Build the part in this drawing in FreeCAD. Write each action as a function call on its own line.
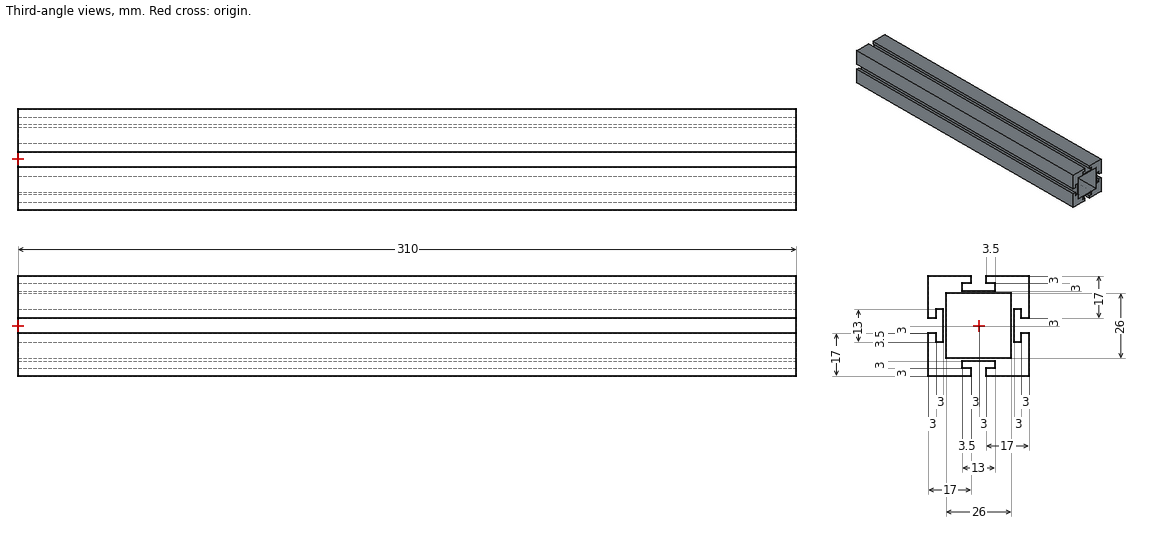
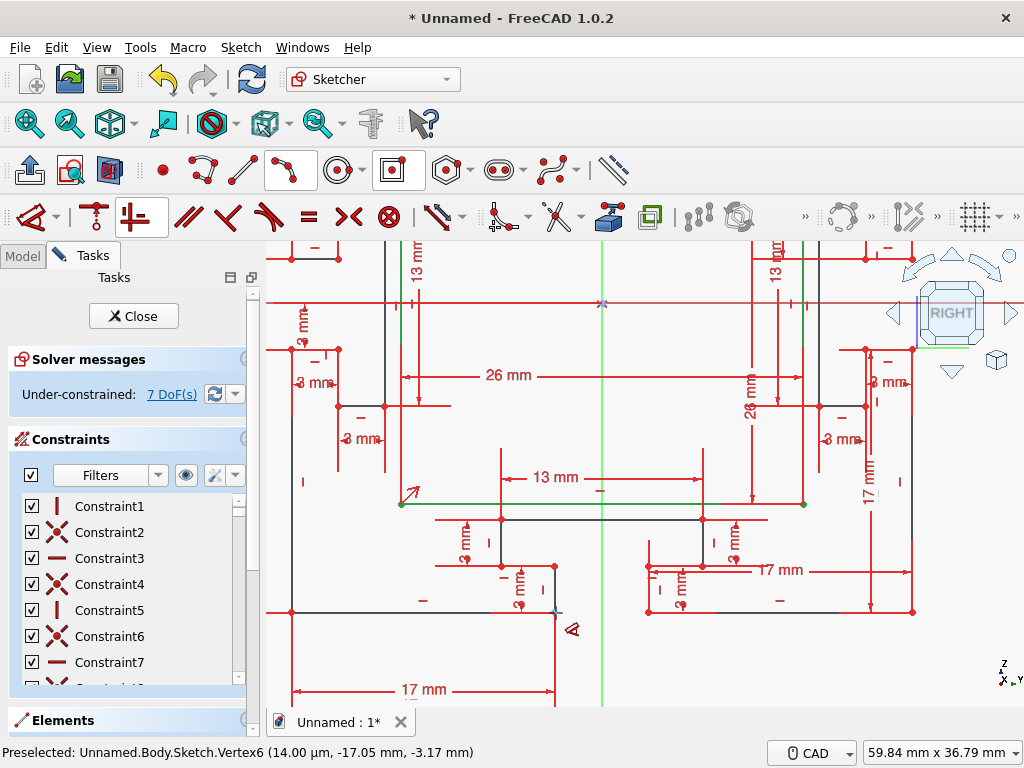
click(555, 613)
click(579, 647)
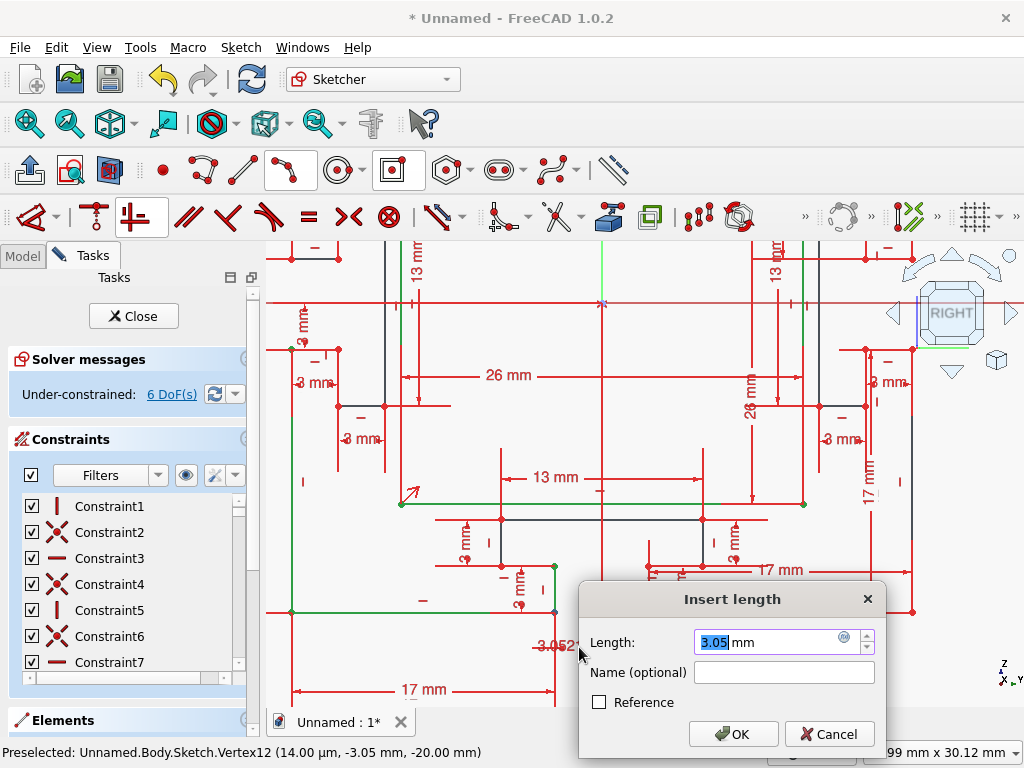
text(3)
key(Return)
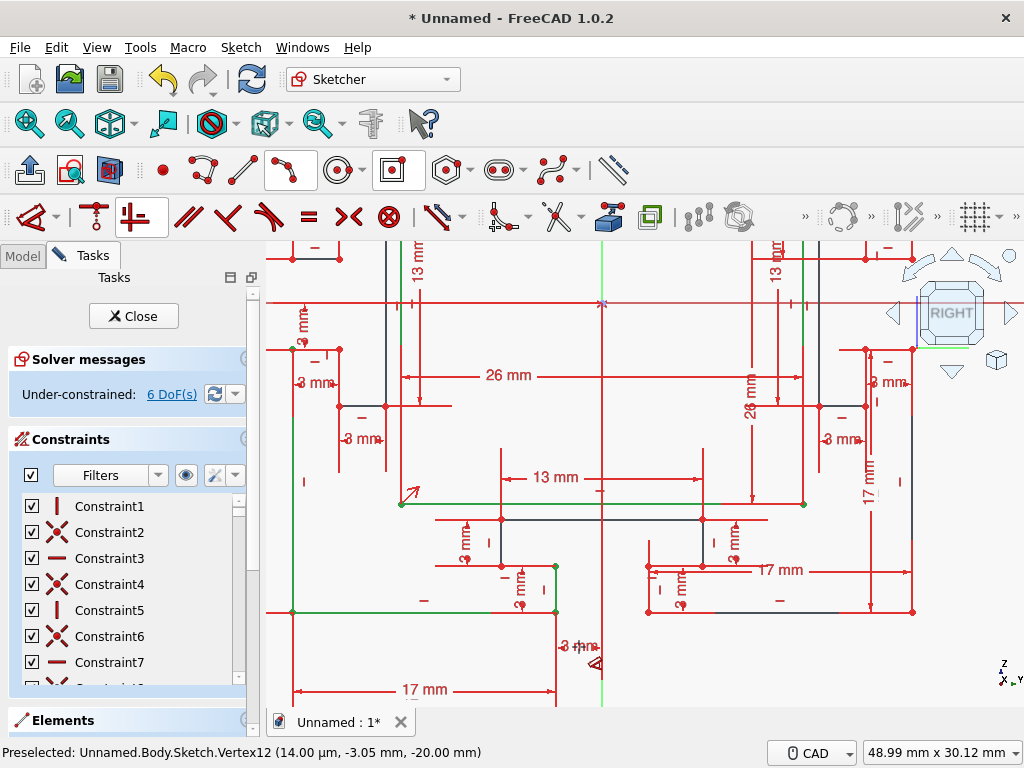
click(649, 566)
click(626, 269)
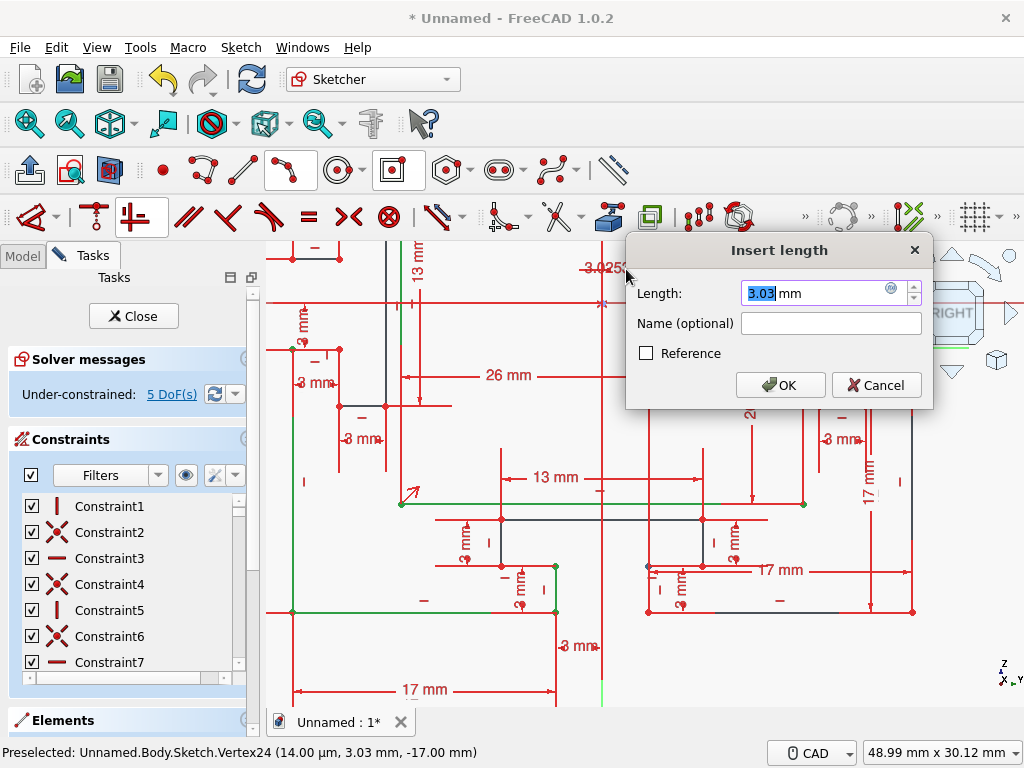
text(3)
key(Return)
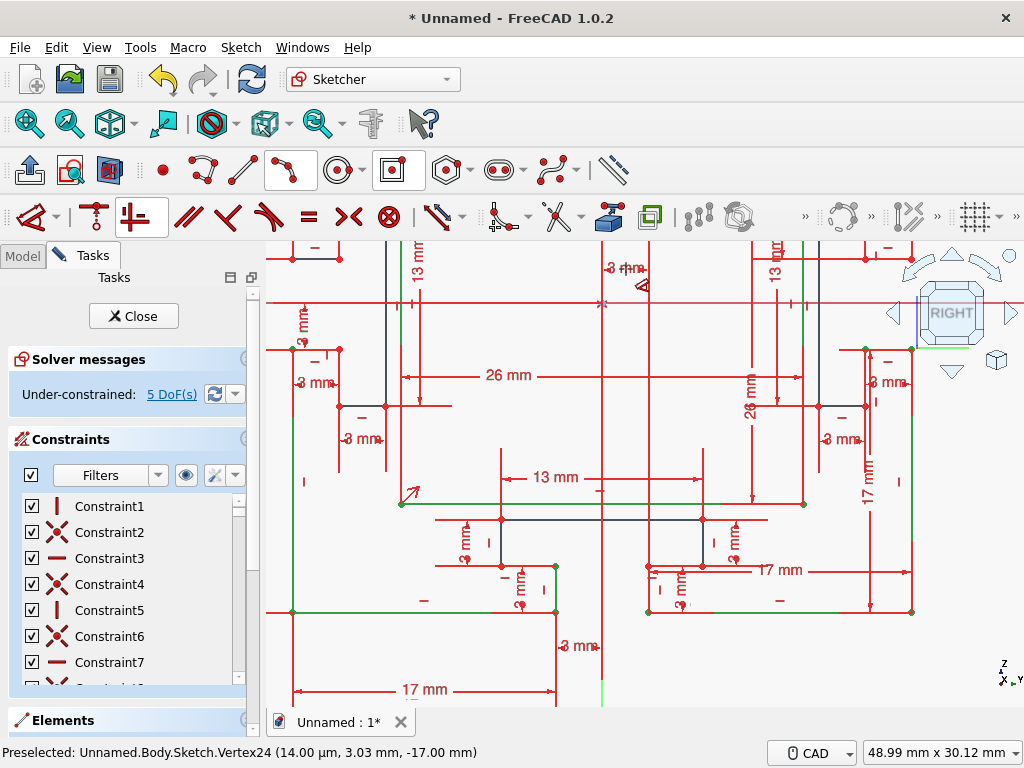
scroll(556, 613, down, 4)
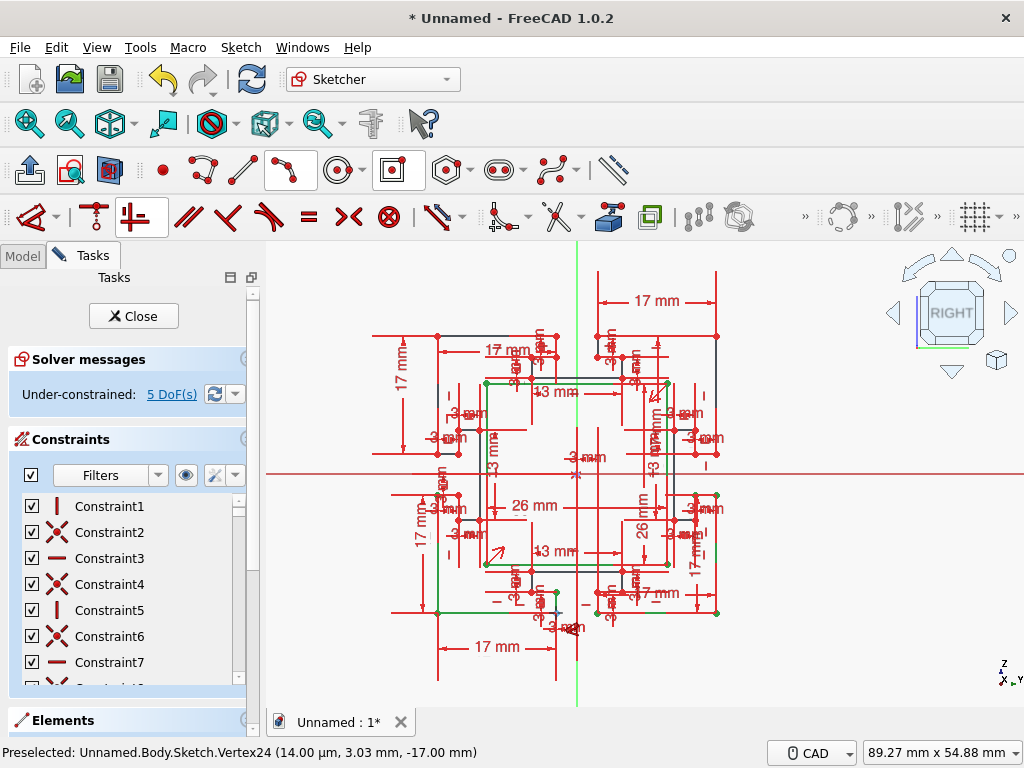
scroll(695, 454, up, 4)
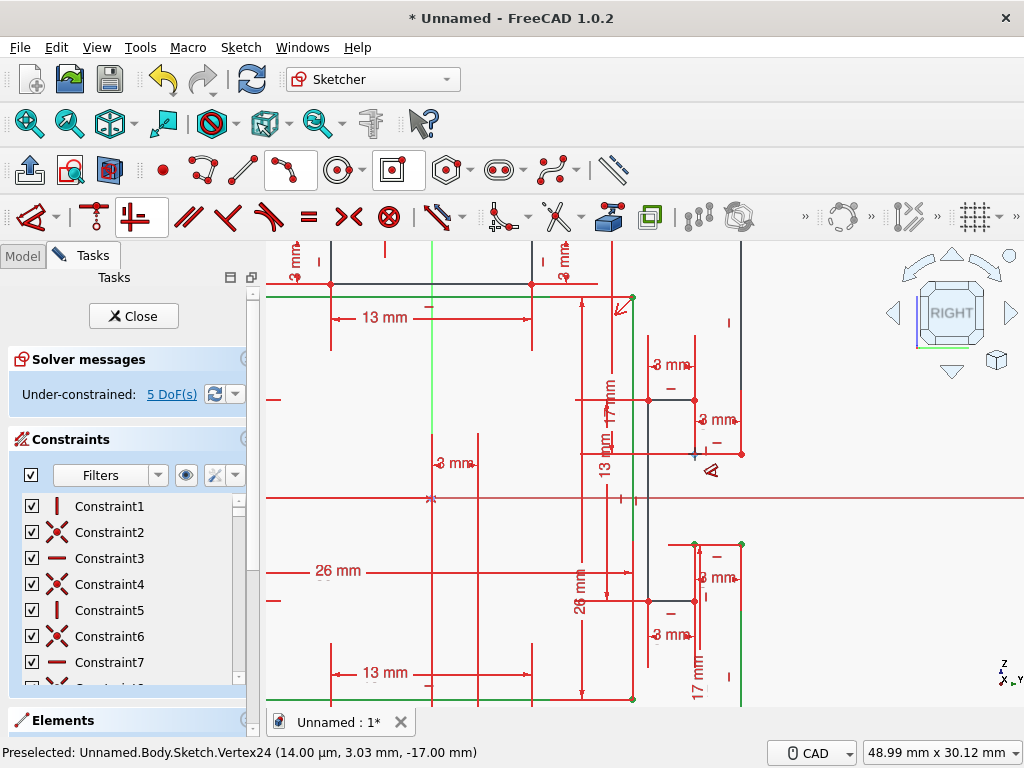
click(695, 454)
click(729, 476)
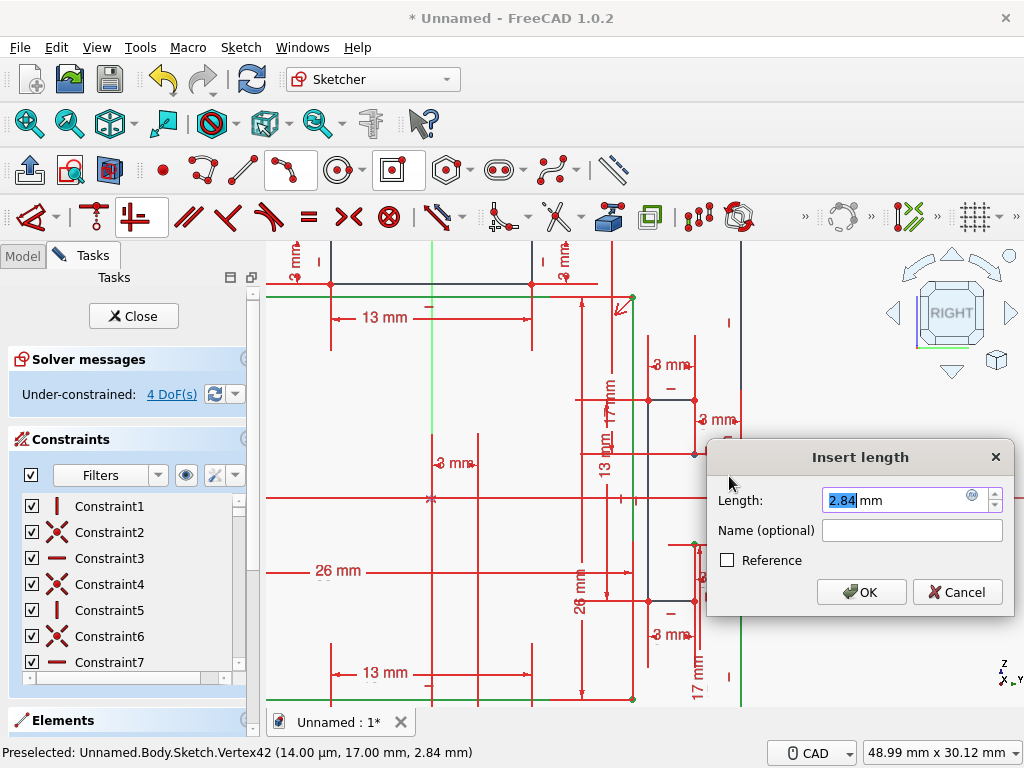
text(3)
key(Return)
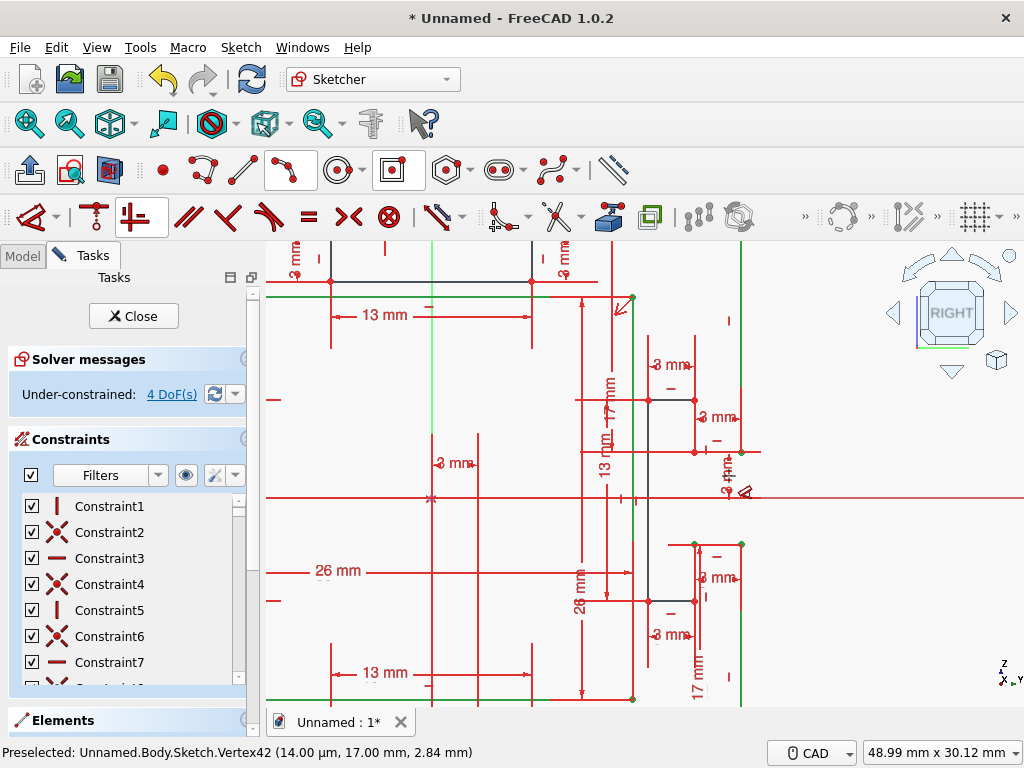
scroll(695, 454, down, 4)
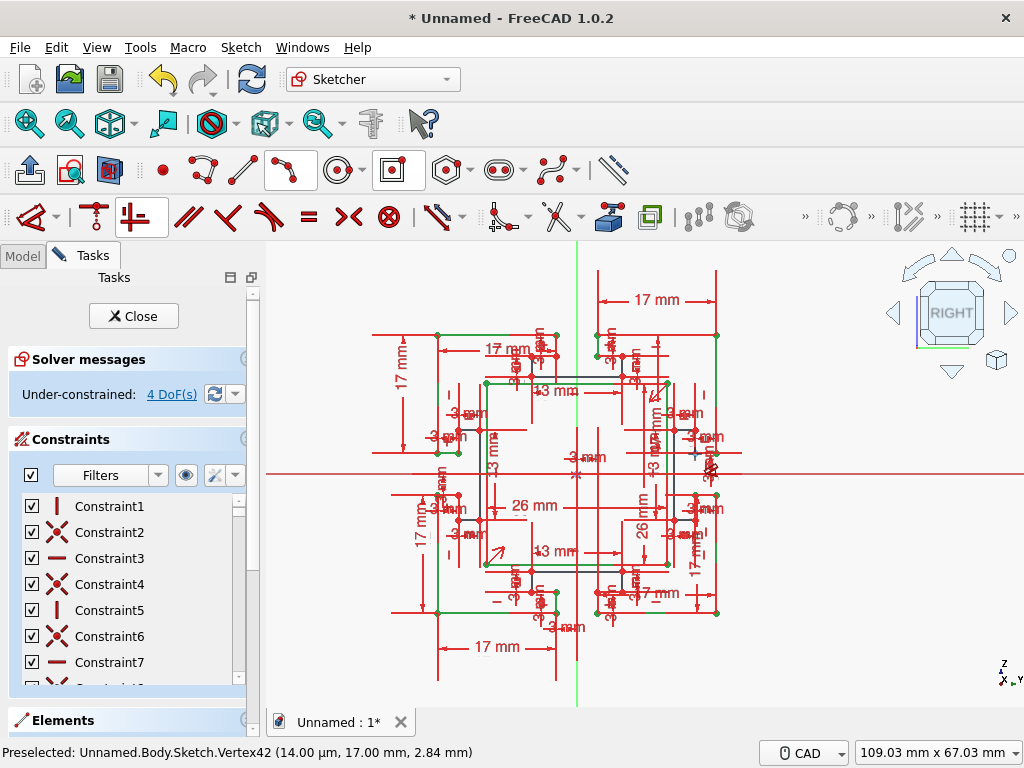
scroll(459, 513, up, 3)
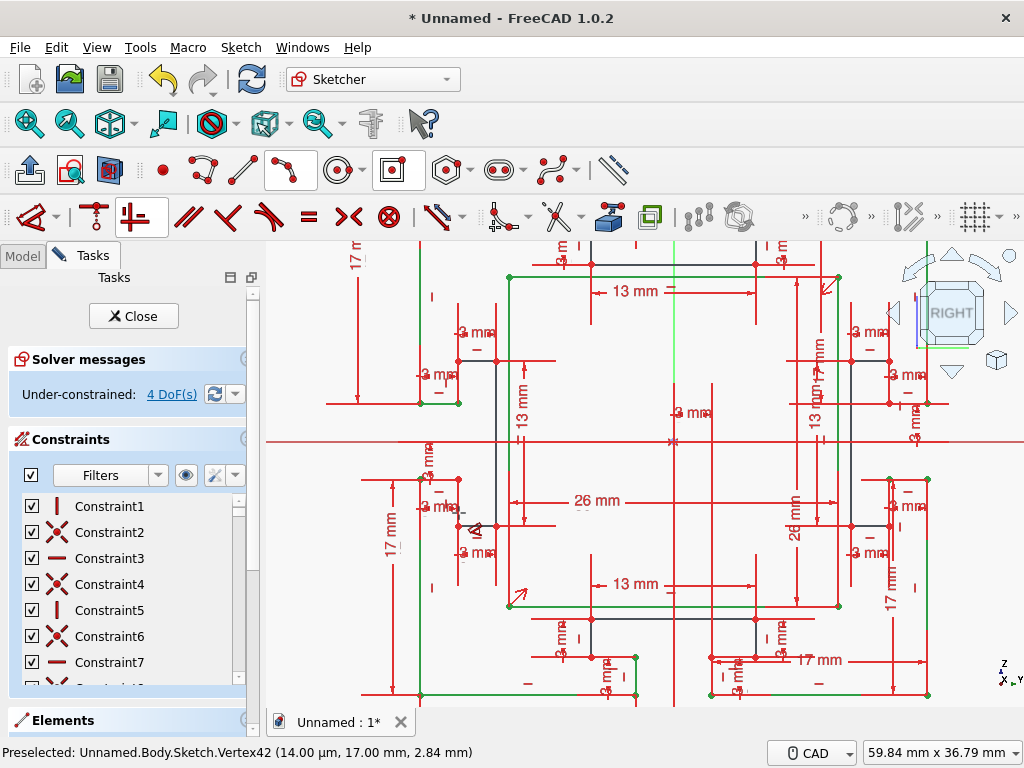
click(458, 512)
click(400, 487)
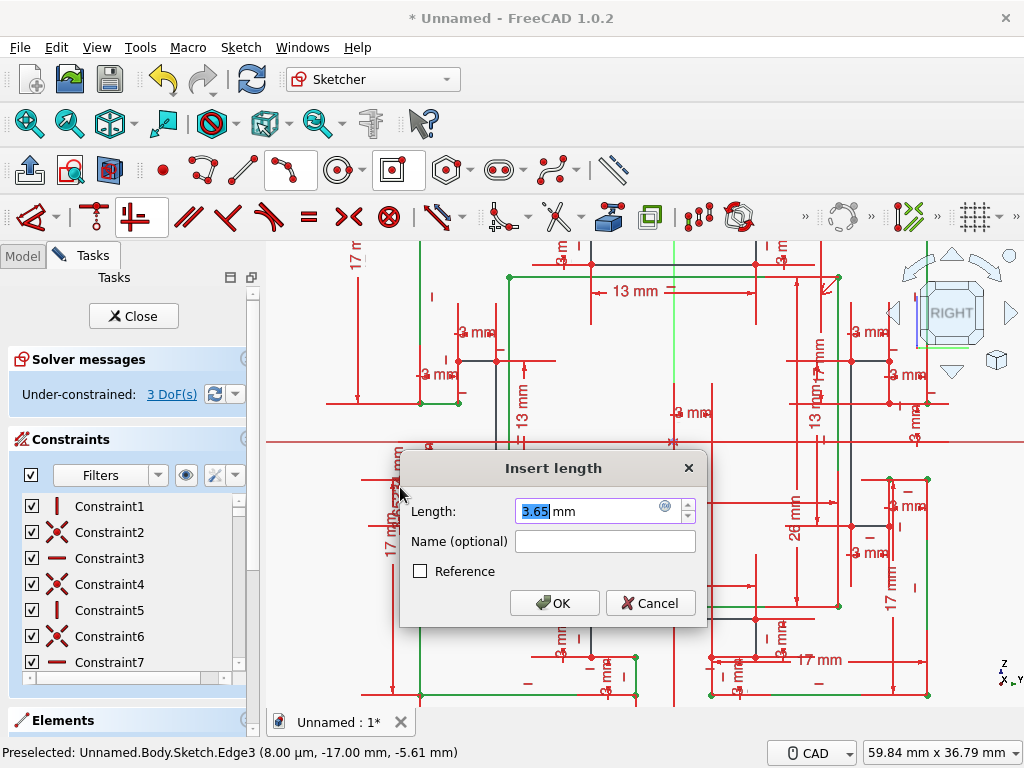
text(3.5)
key(Return)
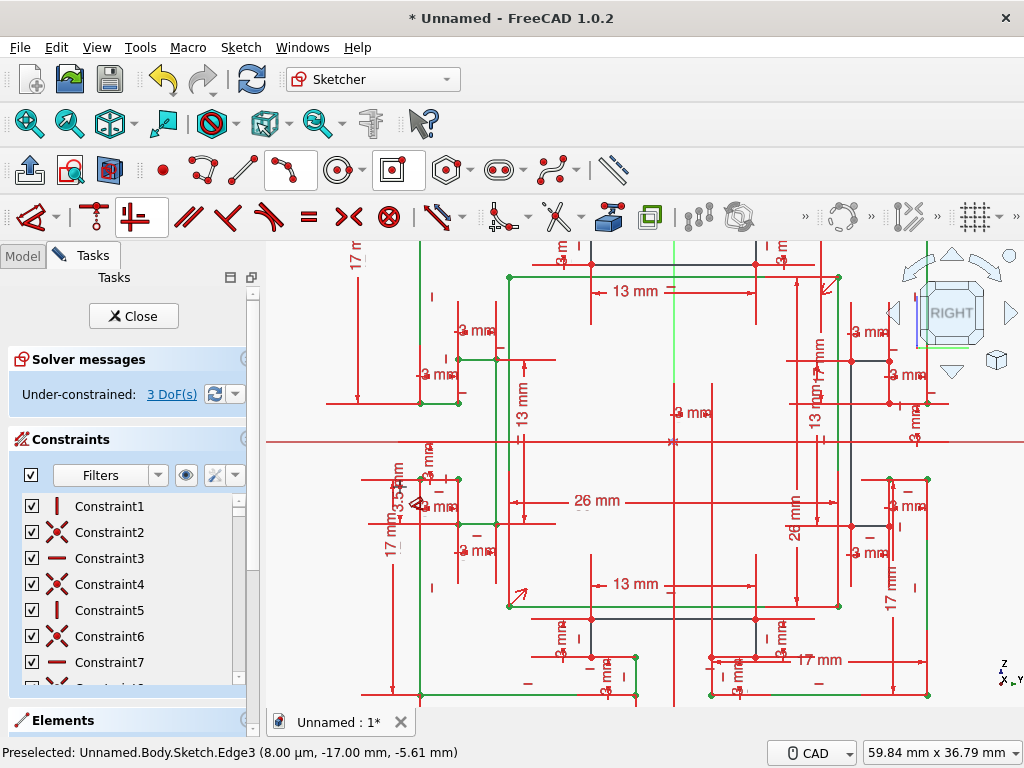
click(622, 657)
click(613, 551)